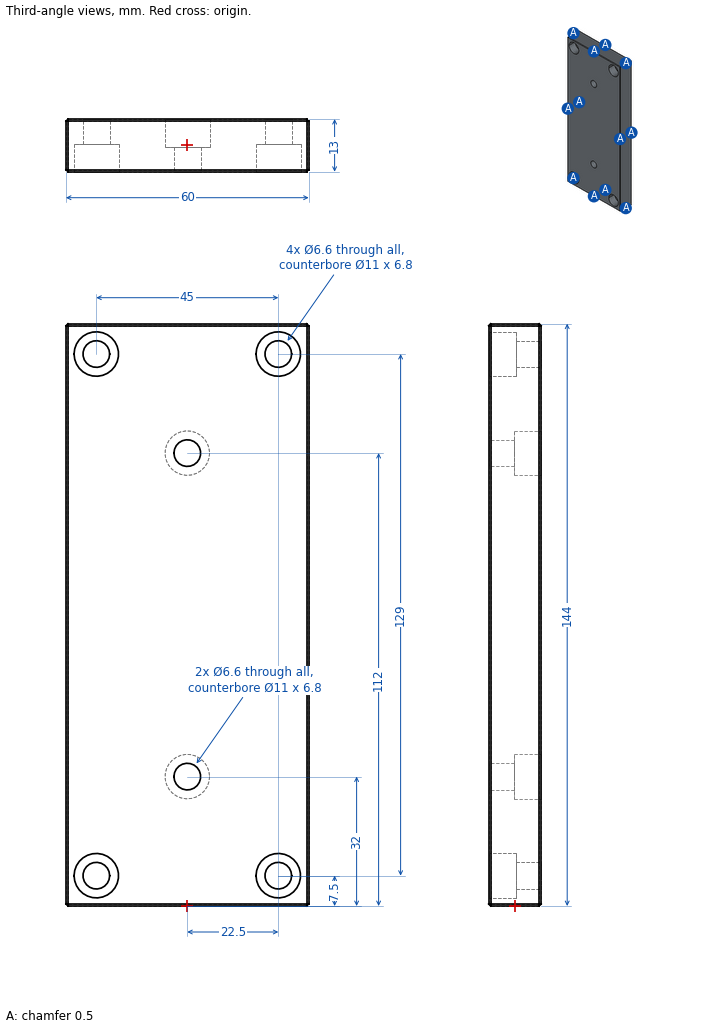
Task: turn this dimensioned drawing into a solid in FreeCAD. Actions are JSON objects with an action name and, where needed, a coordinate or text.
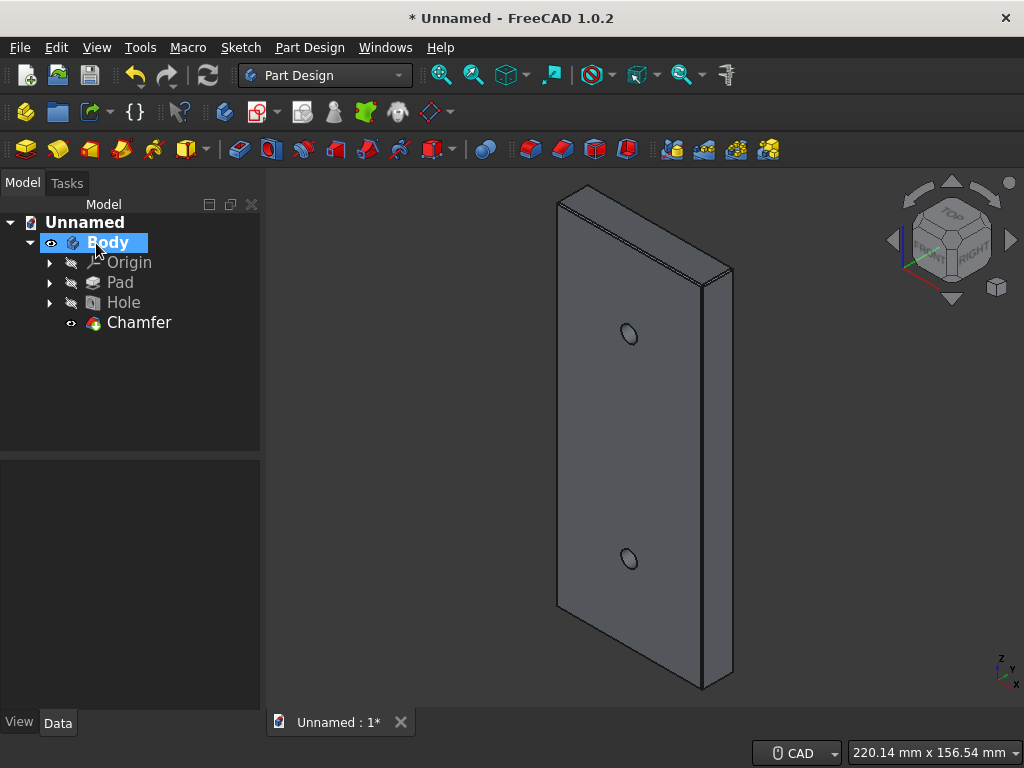
{"action": "left_click", "coordinate": [629, 446]}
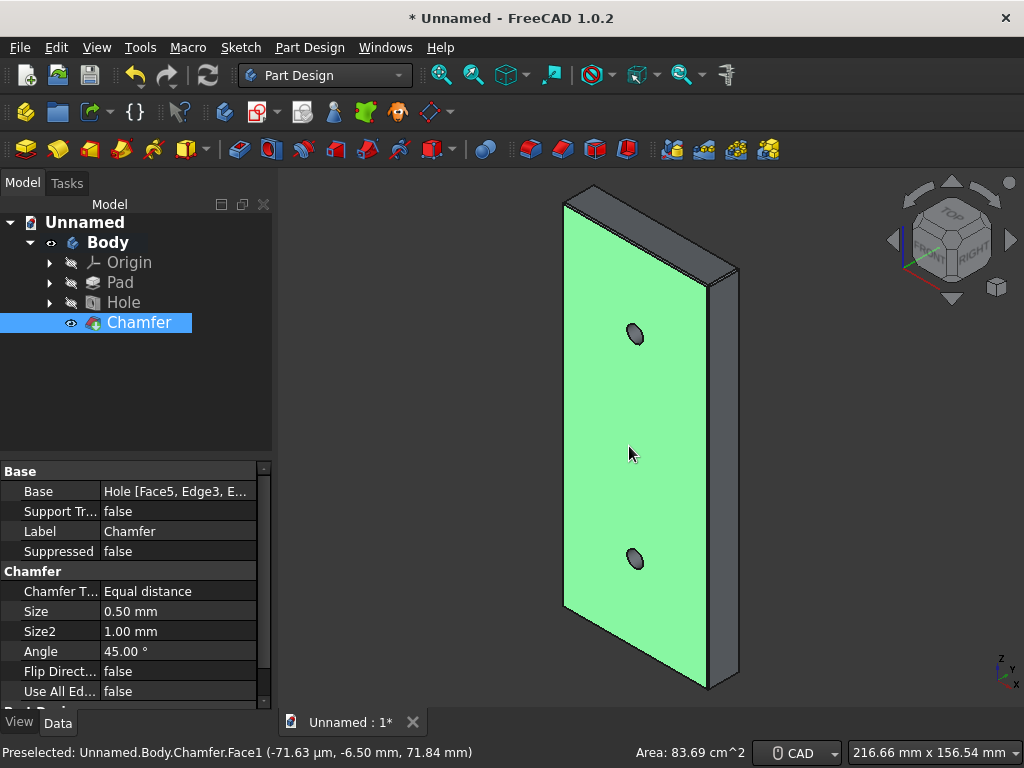
{"action": "left_click", "coordinate": [258, 112]}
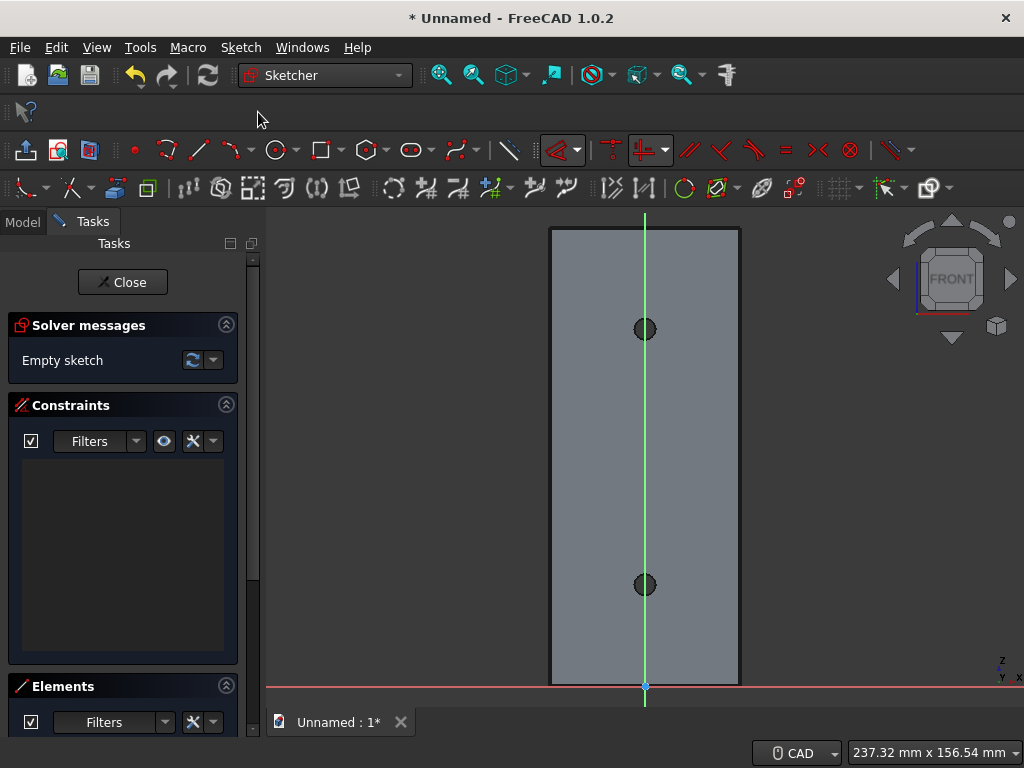
{"action": "scroll", "coordinate": [437, 443], "scroll_direction": "down", "scroll_amount": 2}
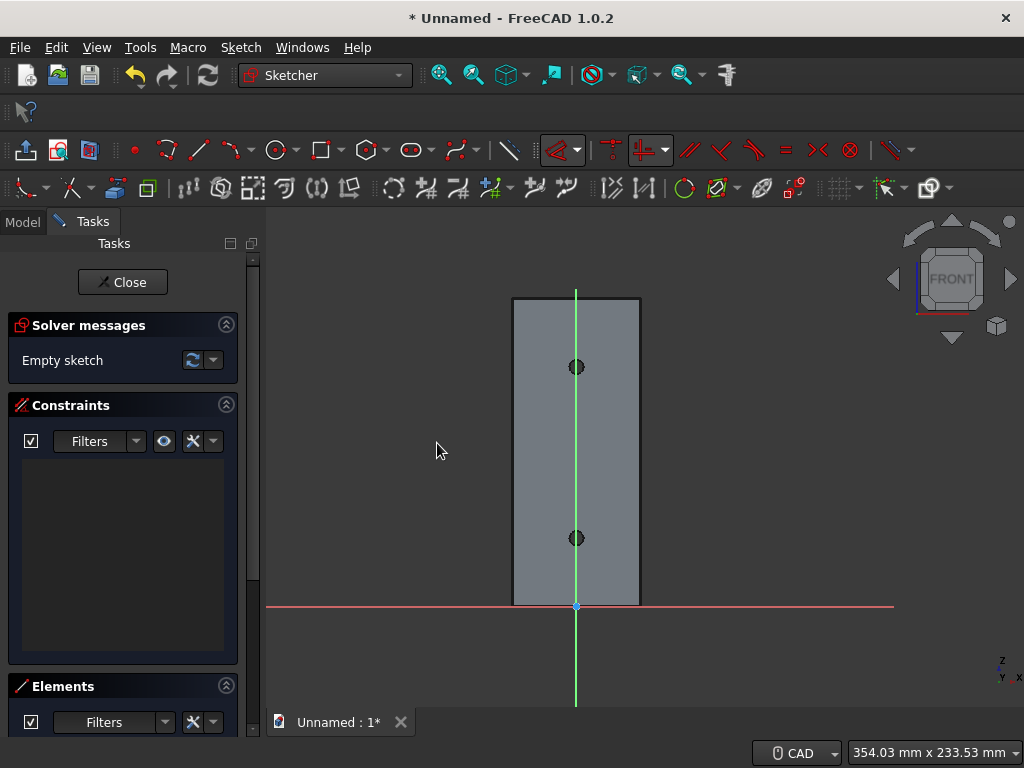
{"action": "key", "text": "g c"}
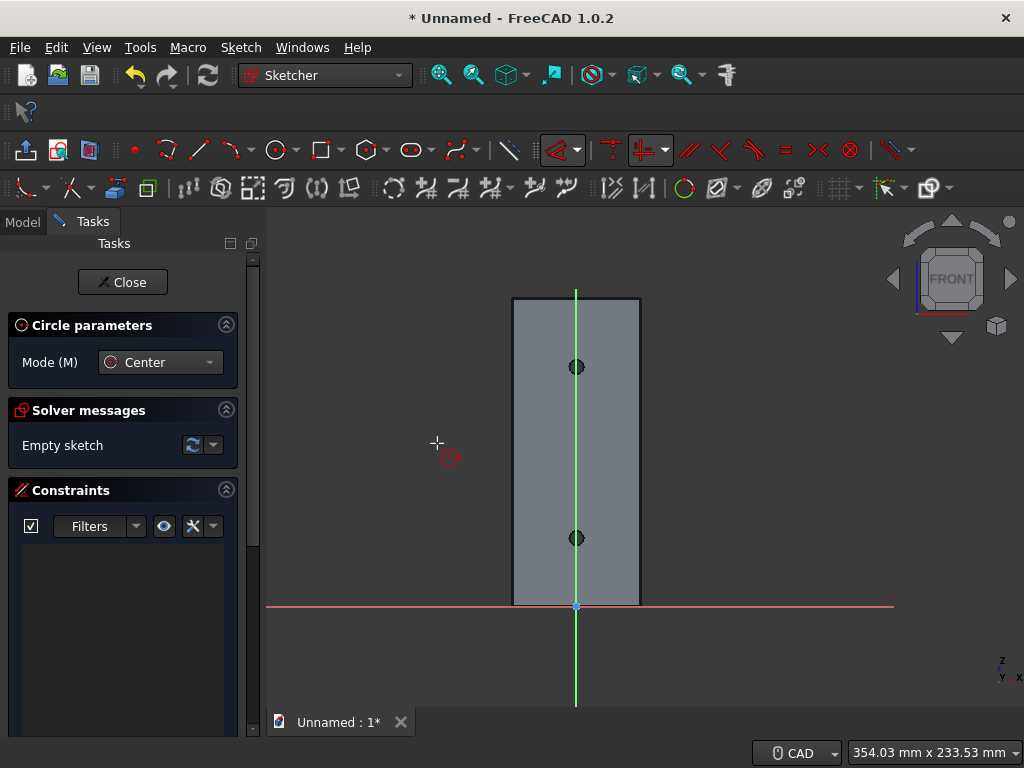
{"action": "scroll", "coordinate": [625, 314], "scroll_direction": "up", "scroll_amount": 6}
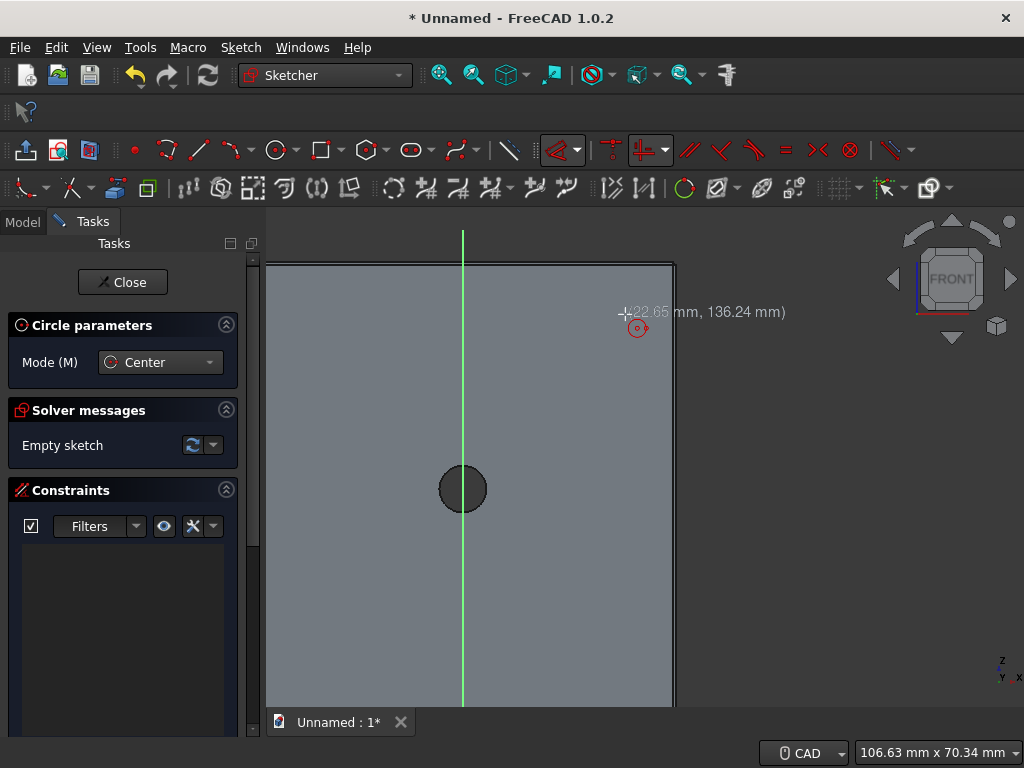
{"action": "left_click", "coordinate": [623, 315]}
{"action": "left_click", "coordinate": [639, 298]}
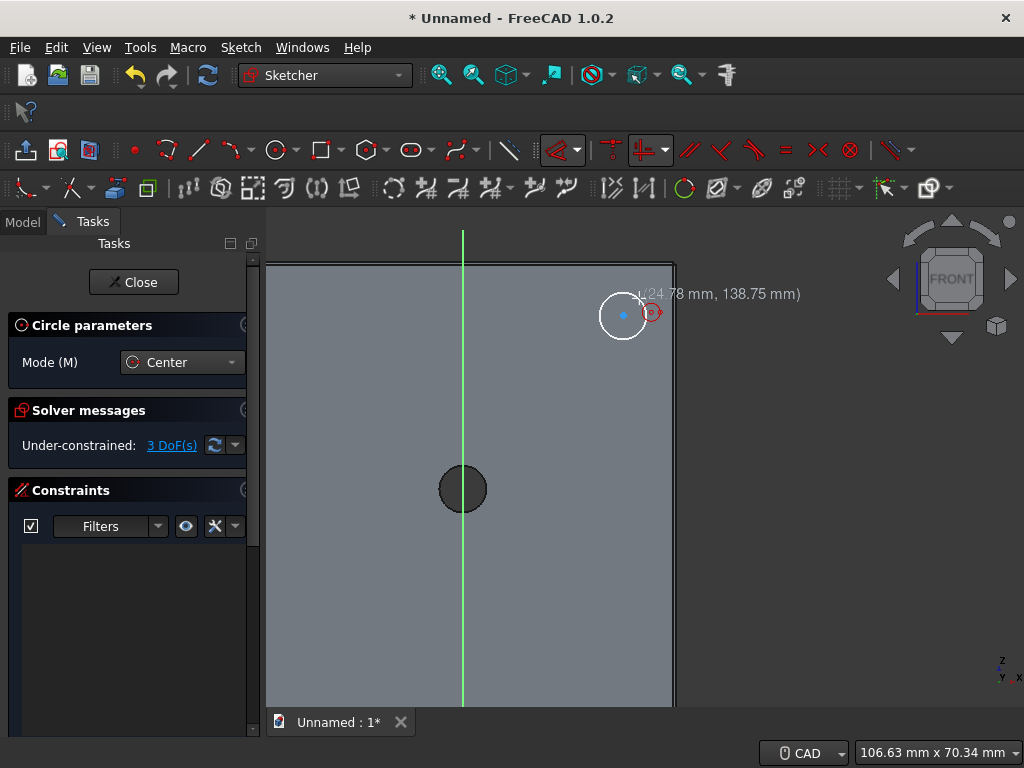
{"action": "left_click", "coordinate": [303, 315]}
{"action": "left_click", "coordinate": [320, 298]}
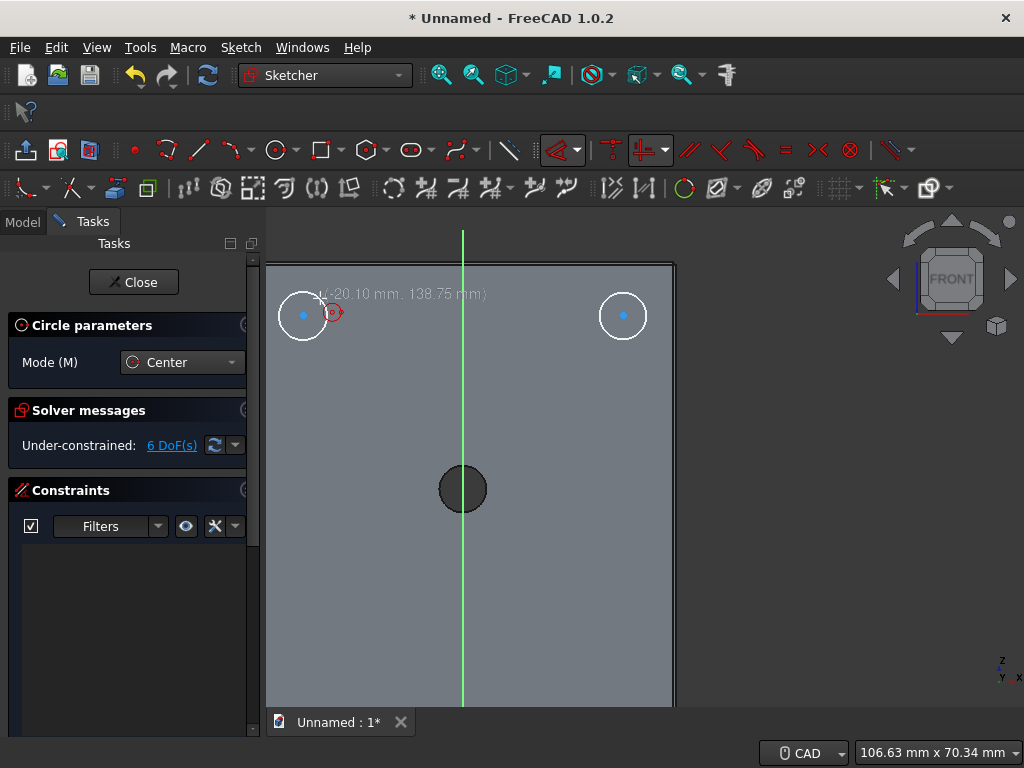
{"action": "scroll", "coordinate": [625, 314], "scroll_direction": "down", "scroll_amount": 6}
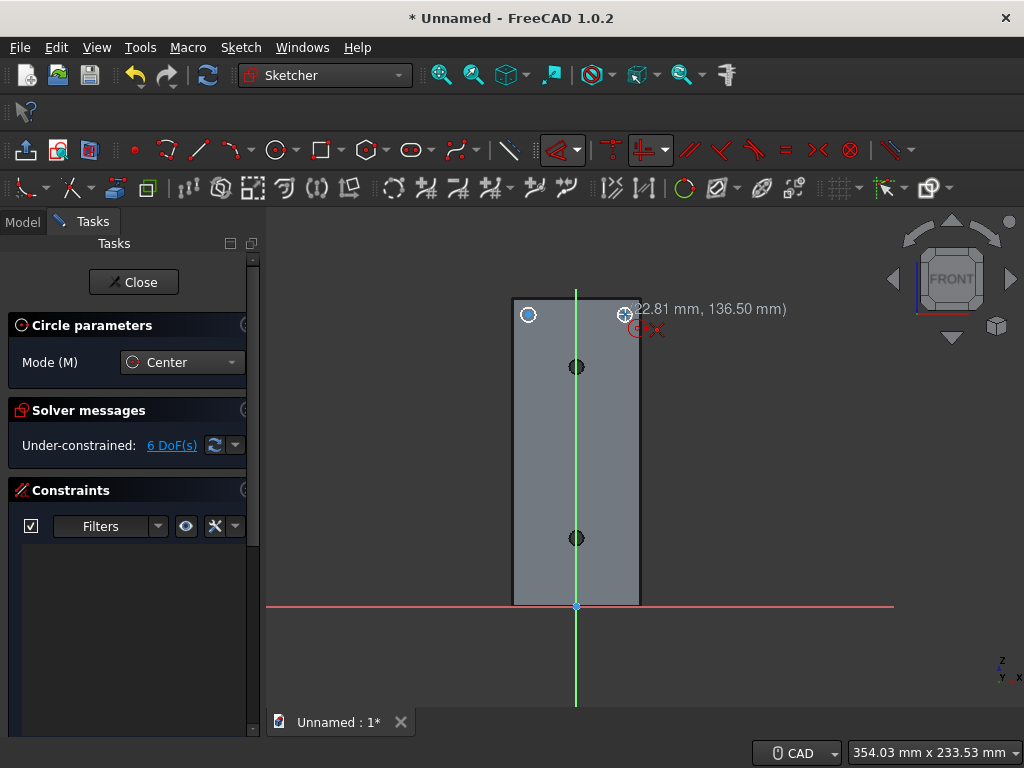
{"action": "scroll", "coordinate": [625, 591], "scroll_direction": "up", "scroll_amount": 6}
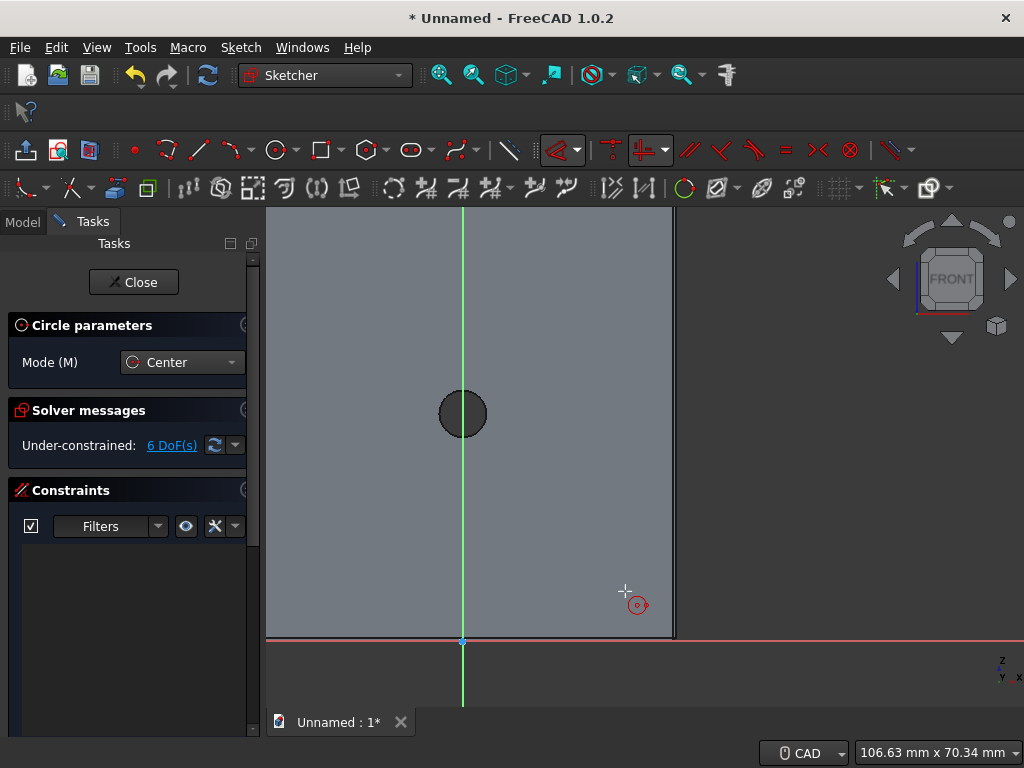
{"action": "left_click", "coordinate": [623, 588]}
{"action": "left_click", "coordinate": [639, 571]}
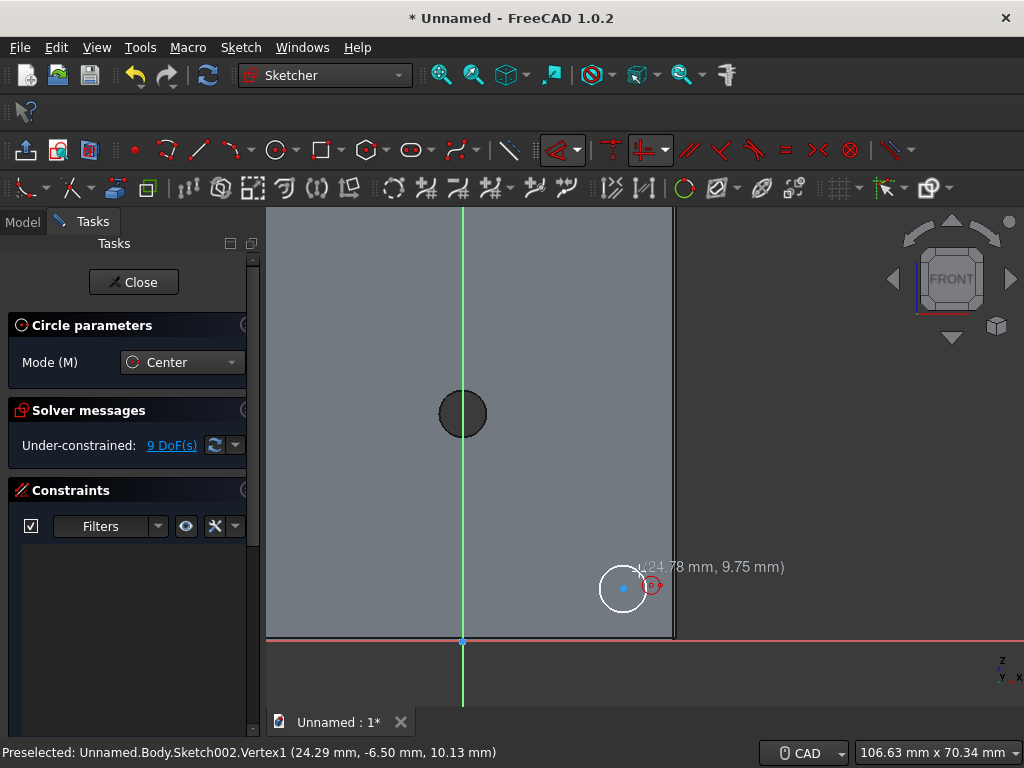
{"action": "left_click", "coordinate": [303, 588]}
{"action": "left_click", "coordinate": [320, 571]}
{"action": "key", "text": "Escape"}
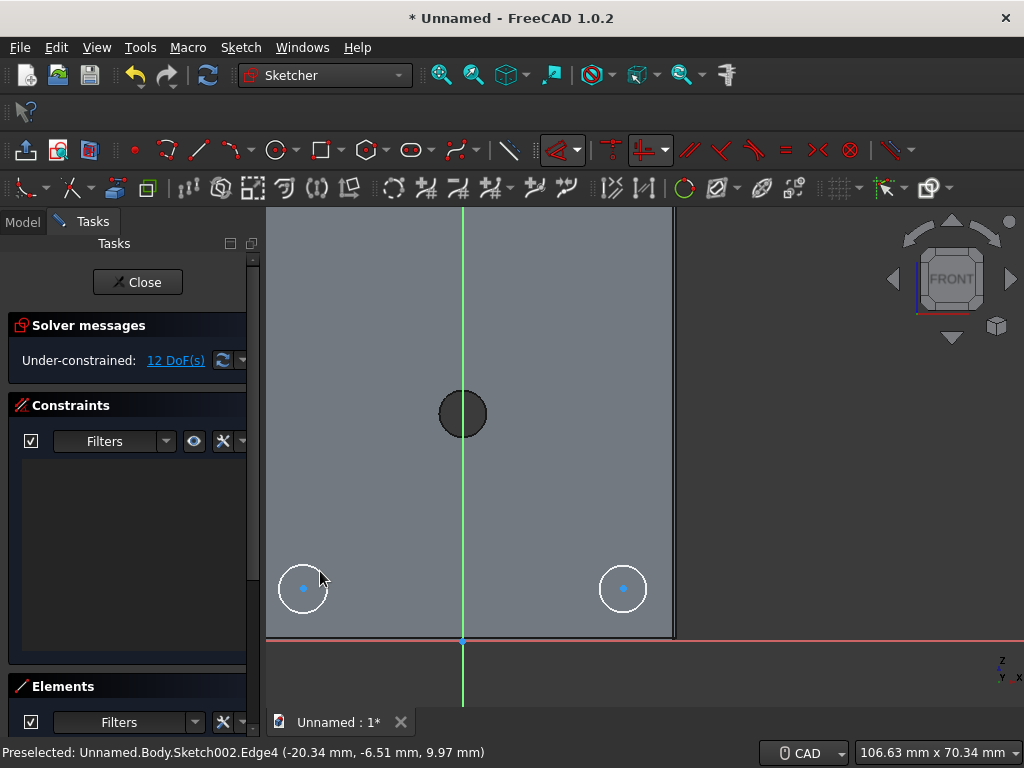
{"action": "scroll", "coordinate": [625, 592], "scroll_direction": "down", "scroll_amount": 6}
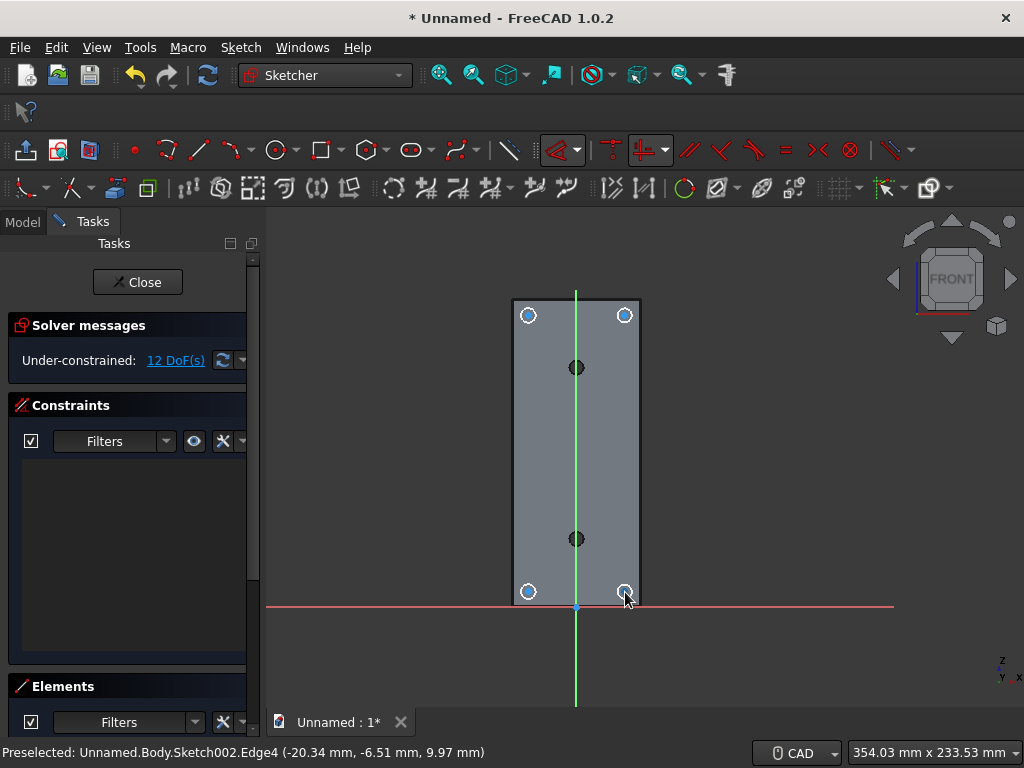
{"action": "scroll", "coordinate": [630, 310], "scroll_direction": "up", "scroll_amount": 4}